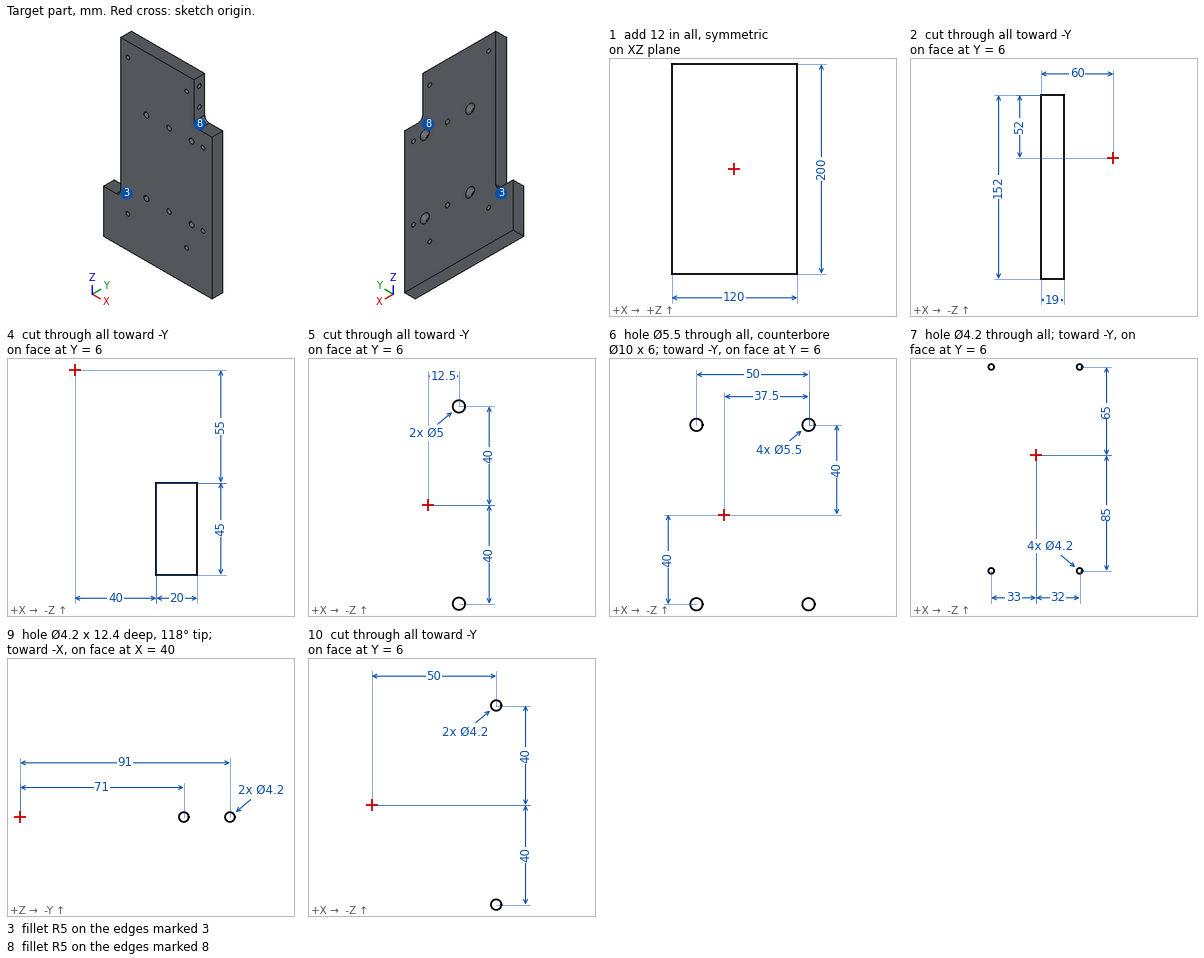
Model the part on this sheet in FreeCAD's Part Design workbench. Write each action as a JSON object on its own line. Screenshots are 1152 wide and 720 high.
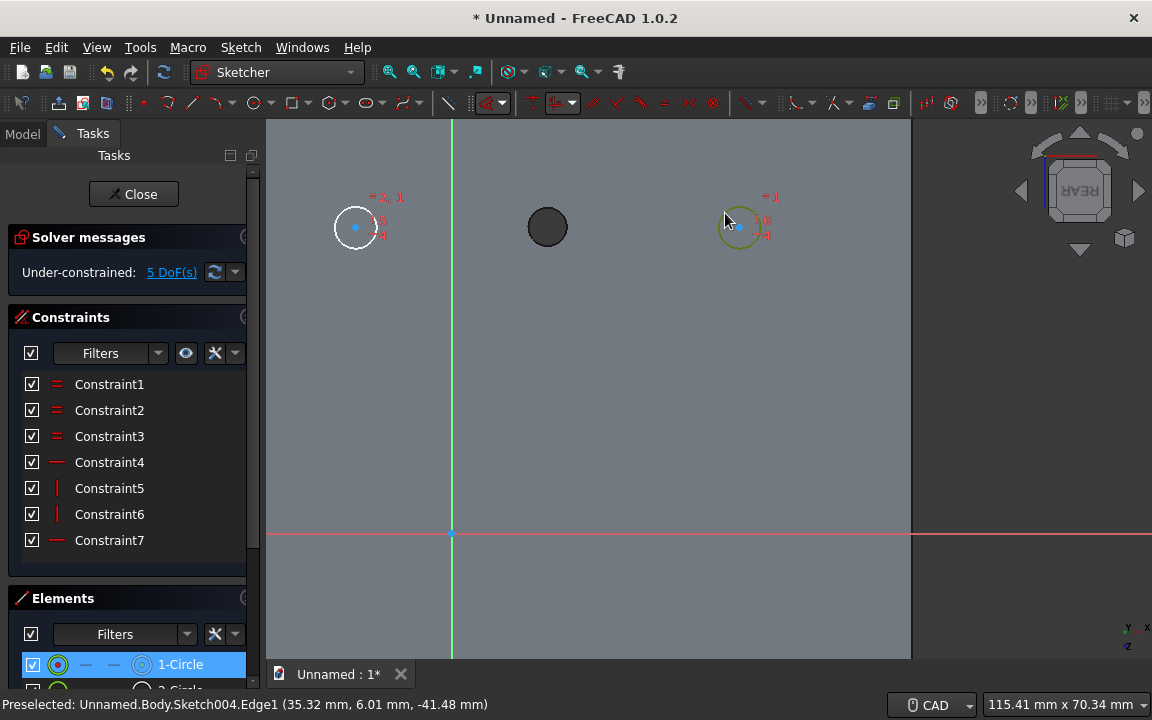
{"action": "left_click", "coordinate": [504, 104]}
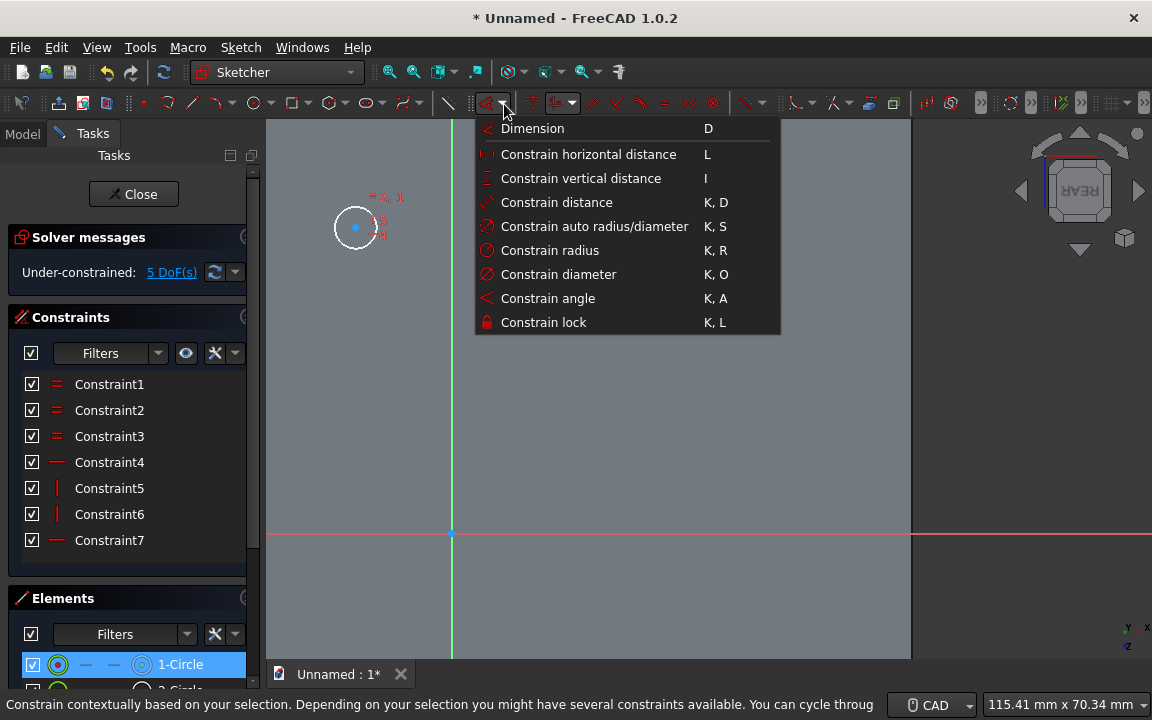
{"action": "left_click", "coordinate": [628, 274]}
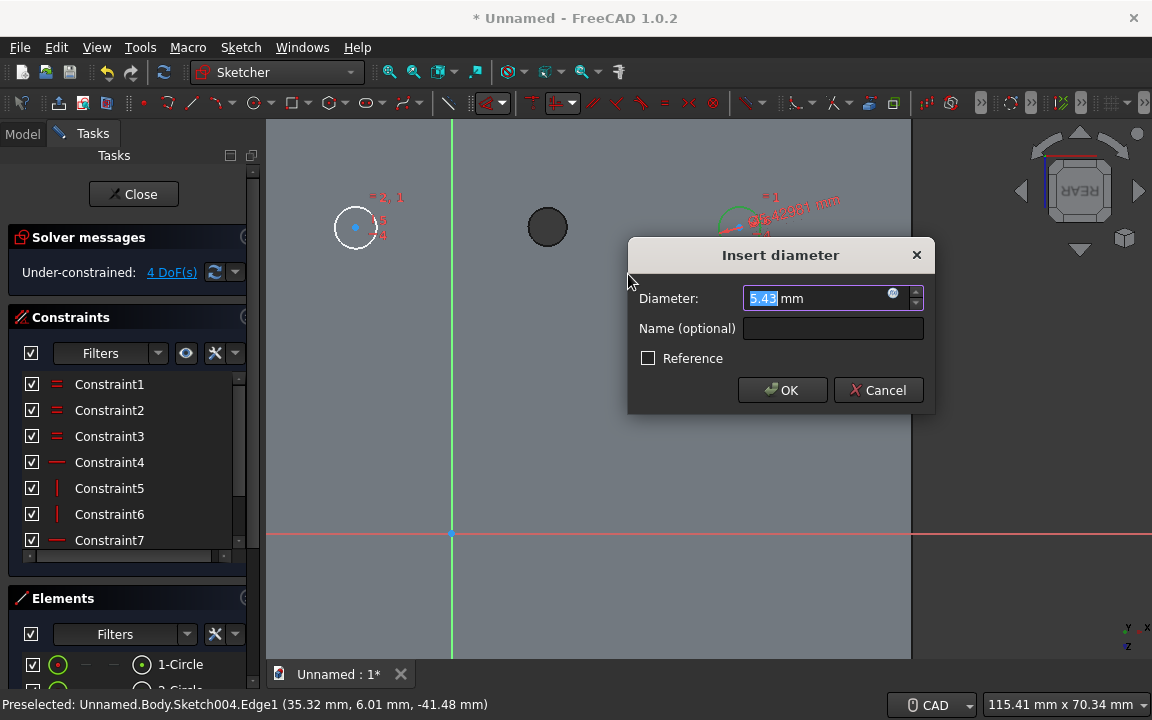
{"action": "type", "text": "5.5"}
{"action": "key", "text": "Return"}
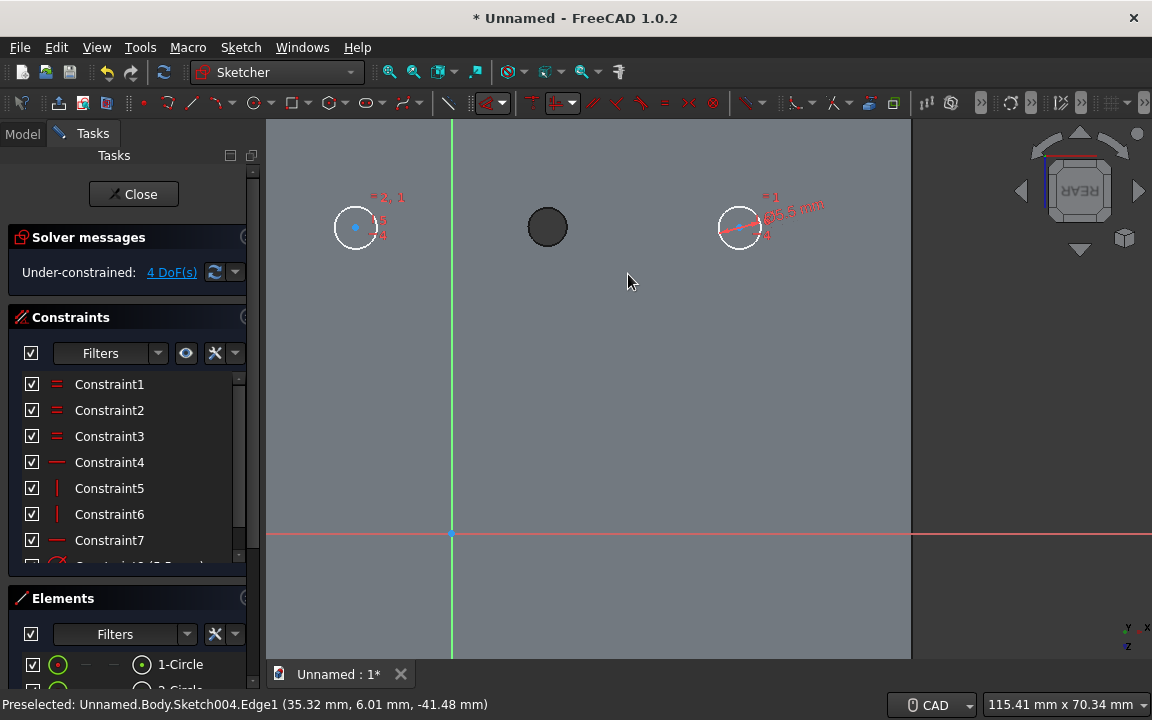
{"action": "left_click", "coordinate": [740, 228]}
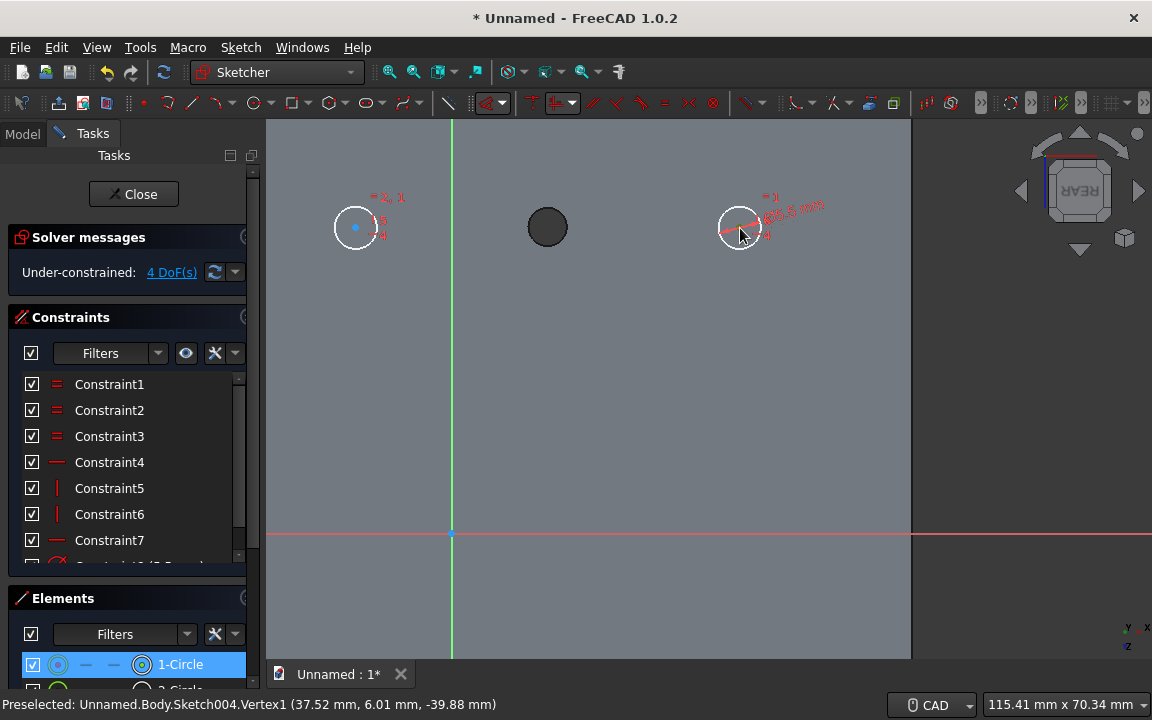
{"action": "left_click", "coordinate": [504, 104]}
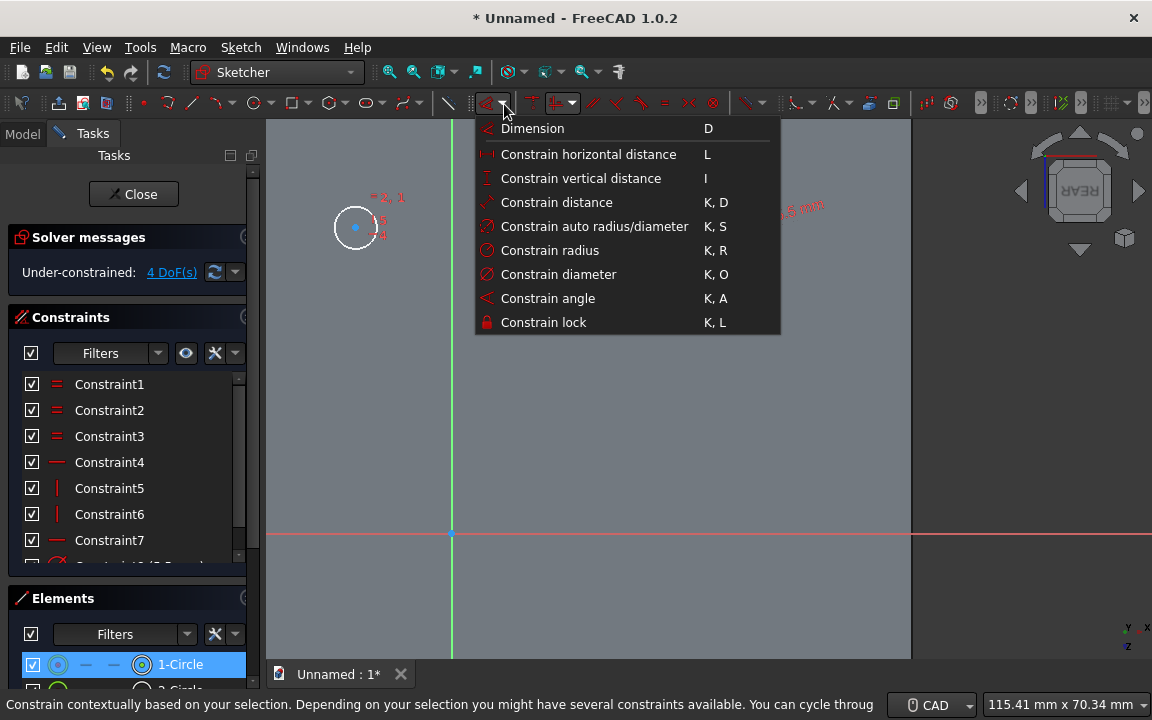
{"action": "left_click", "coordinate": [628, 178]}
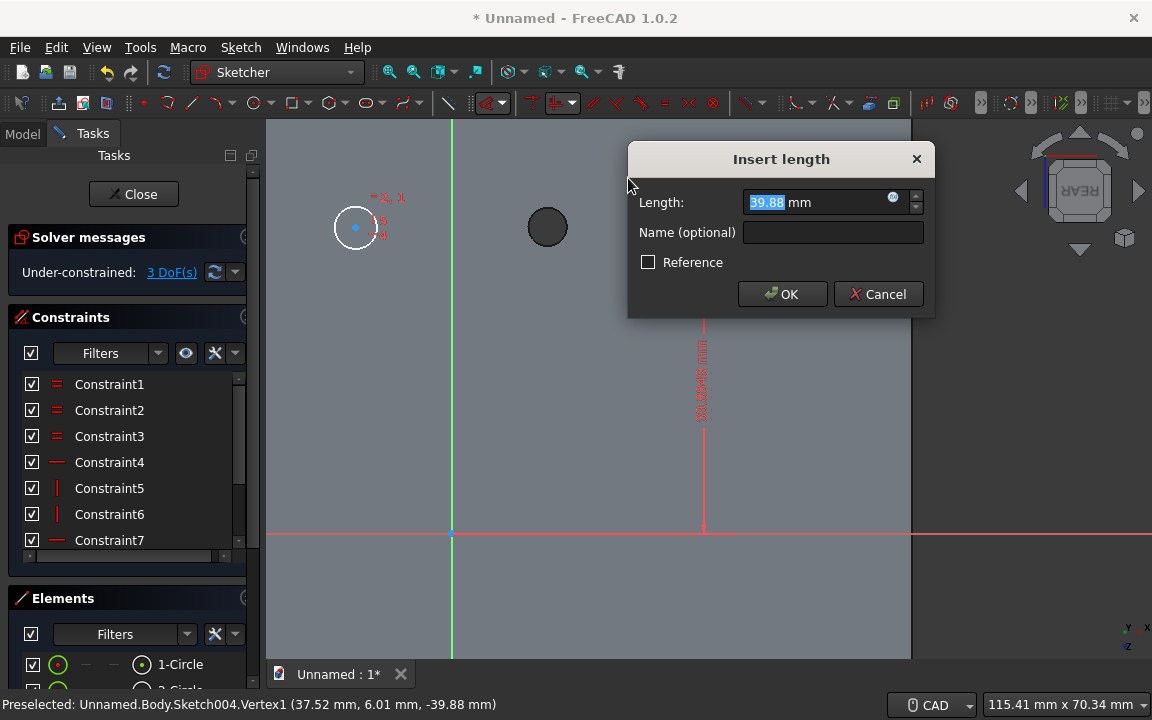
{"action": "type", "text": "40"}
{"action": "key", "text": "Return"}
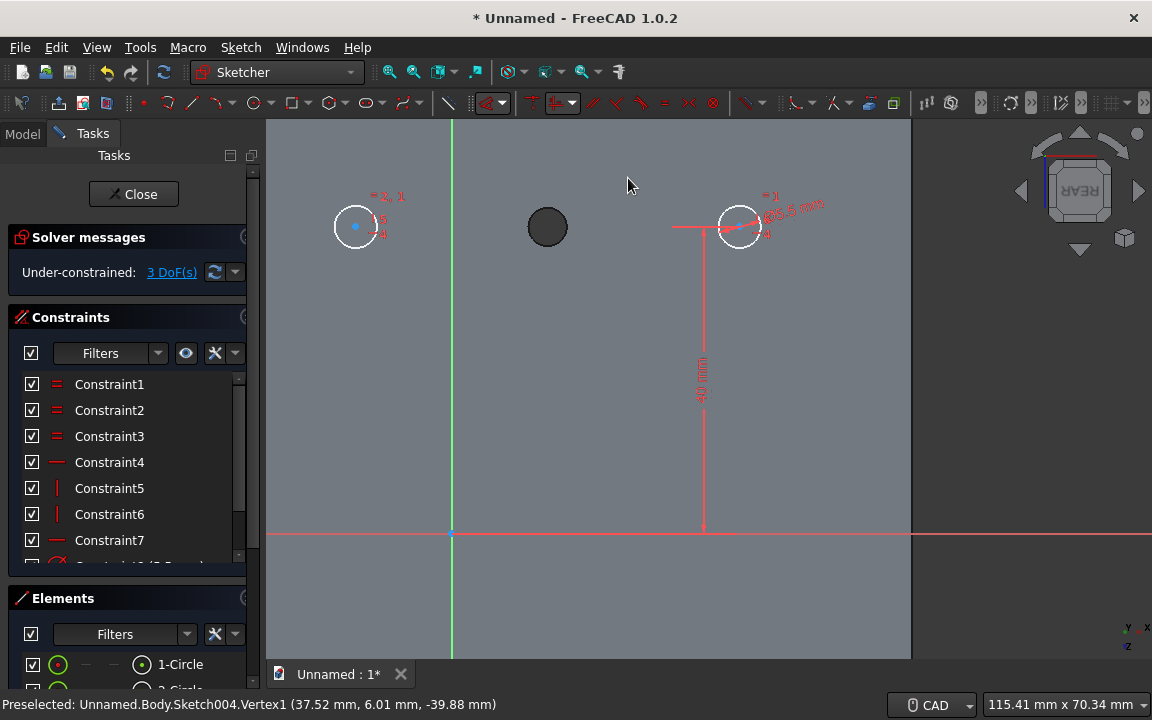
{"action": "scroll", "coordinate": [753, 213], "scroll_direction": "down", "scroll_amount": 3}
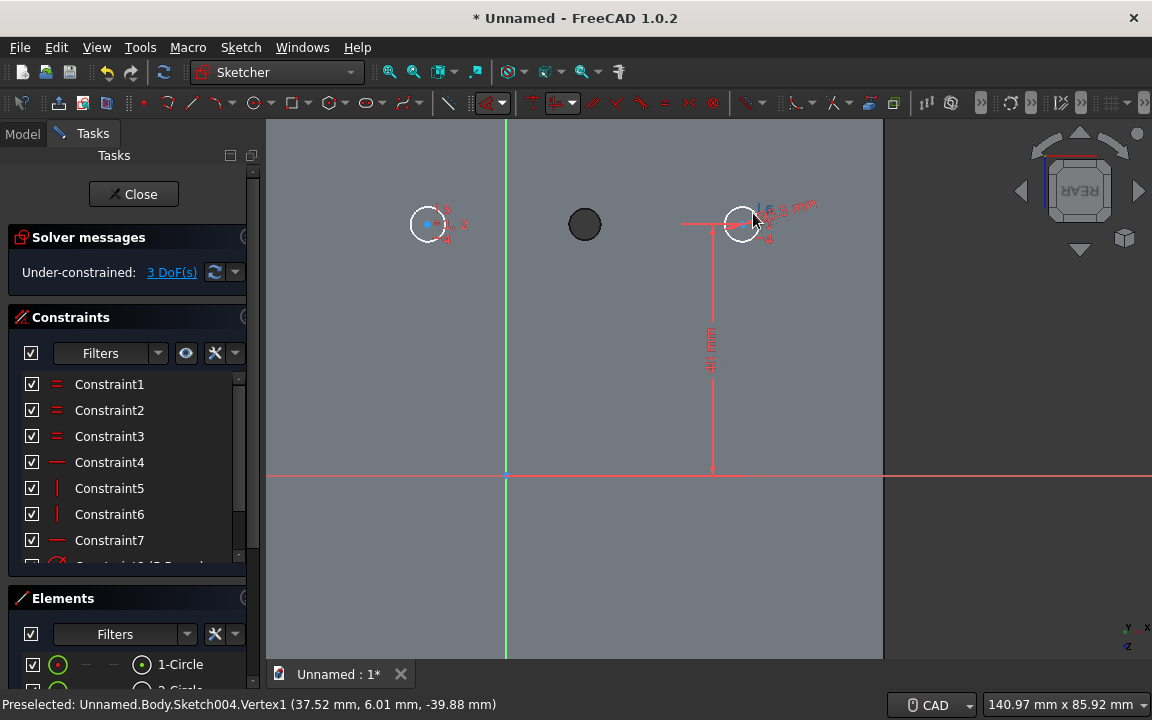
{"action": "left_click", "coordinate": [535, 558]}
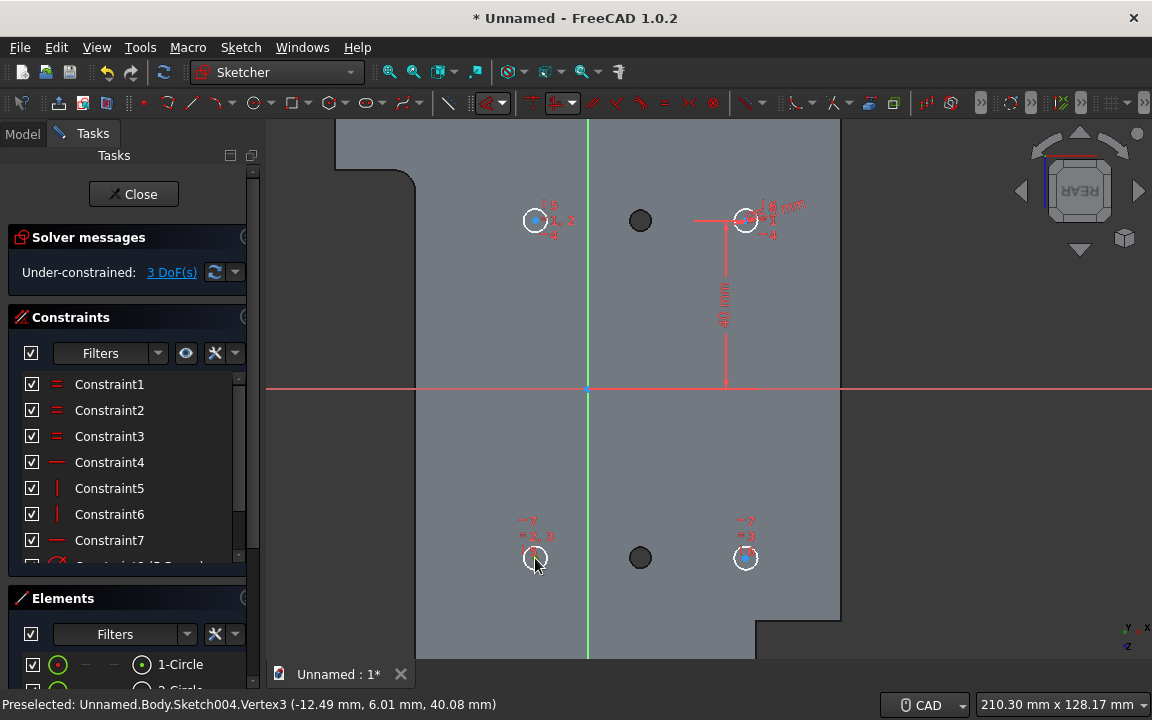
{"action": "key", "text": "i"}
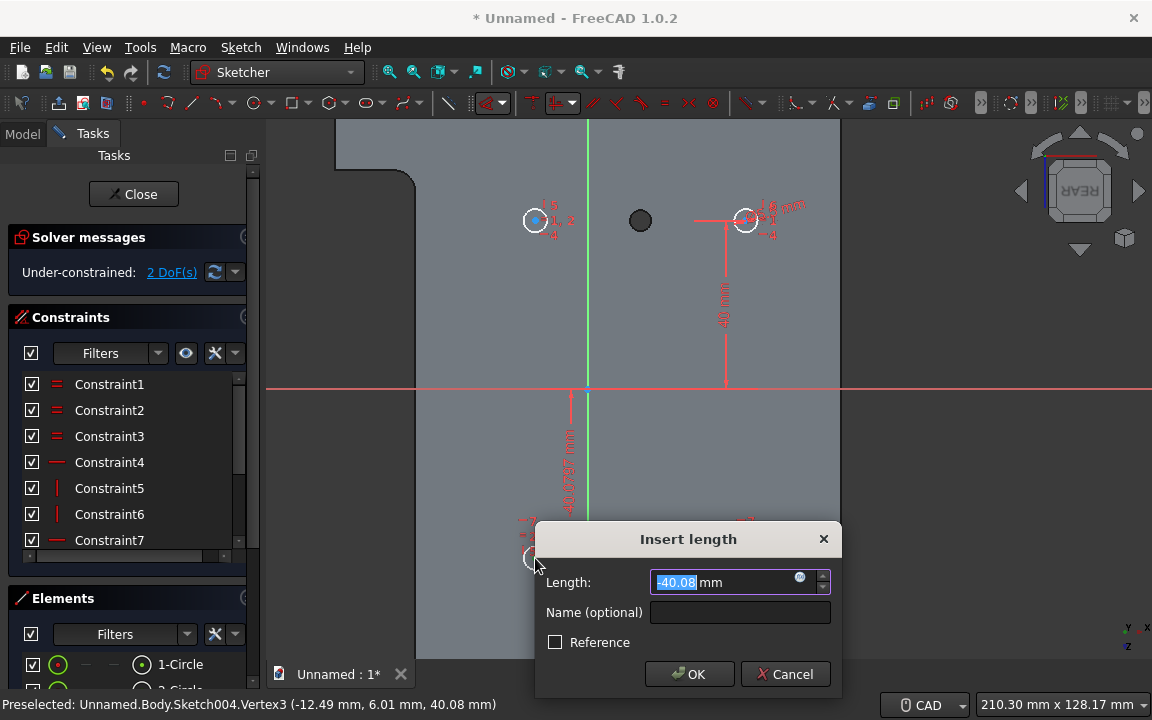
{"action": "type", "text": "-40"}
{"action": "key", "text": "Return"}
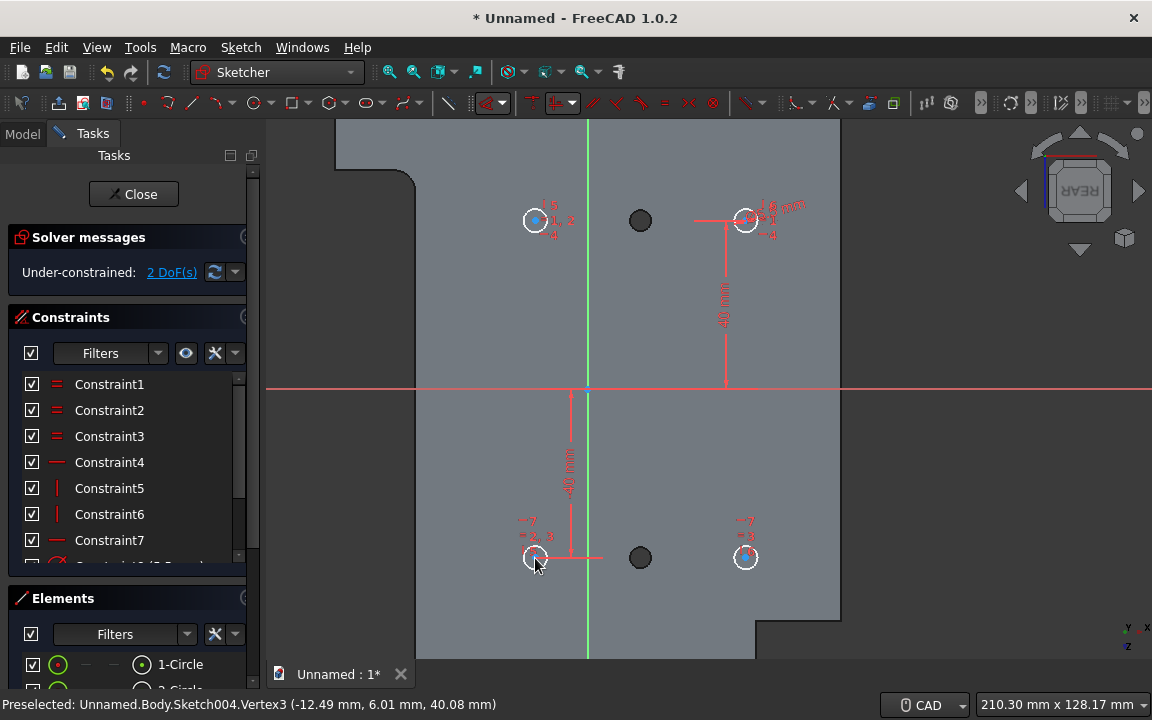
{"action": "left_click", "coordinate": [746, 221]}